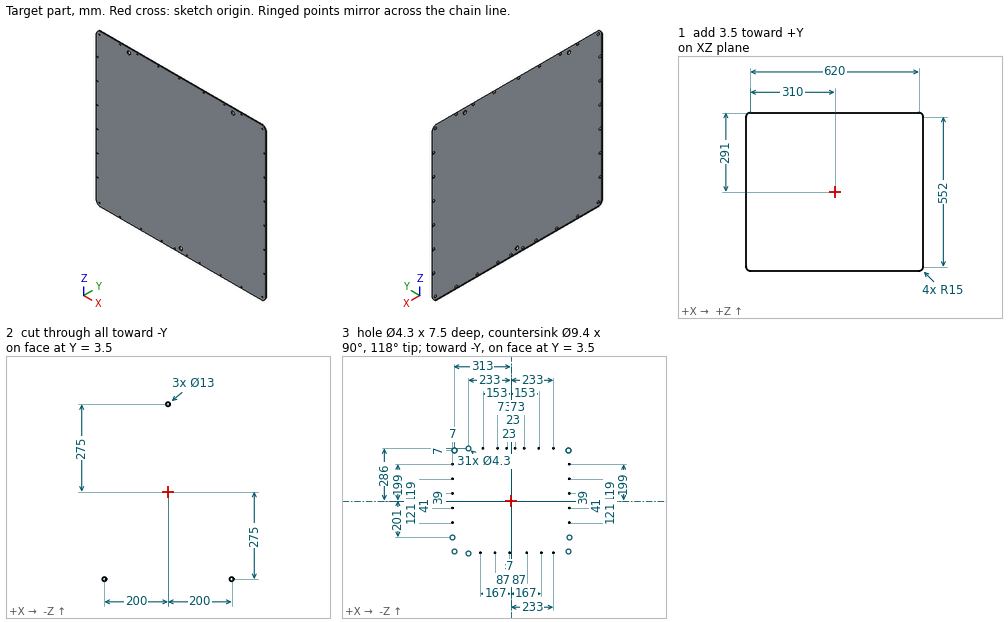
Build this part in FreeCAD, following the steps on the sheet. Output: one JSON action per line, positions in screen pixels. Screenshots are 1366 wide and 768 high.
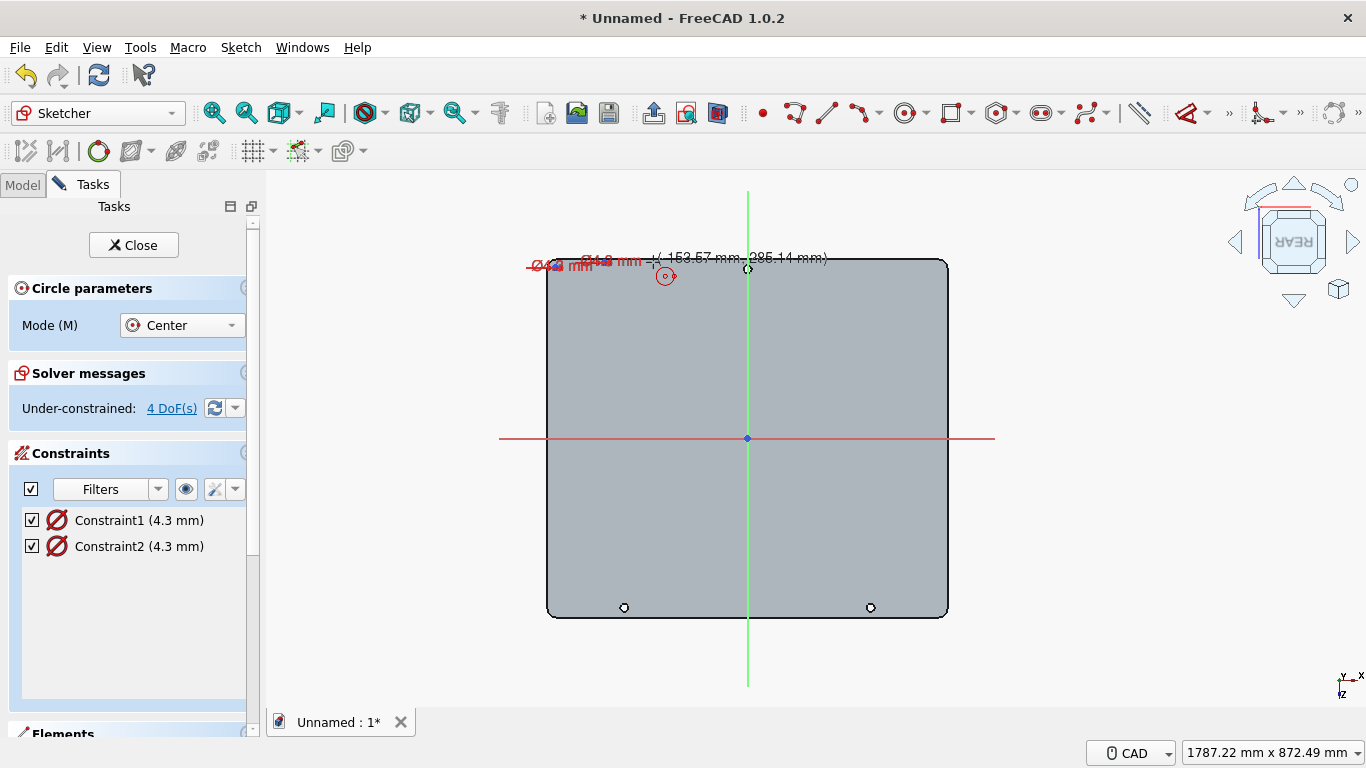
{"action": "left_click", "coordinate": [653, 262]}
{"action": "mouse_move", "coordinate": [654, 262]}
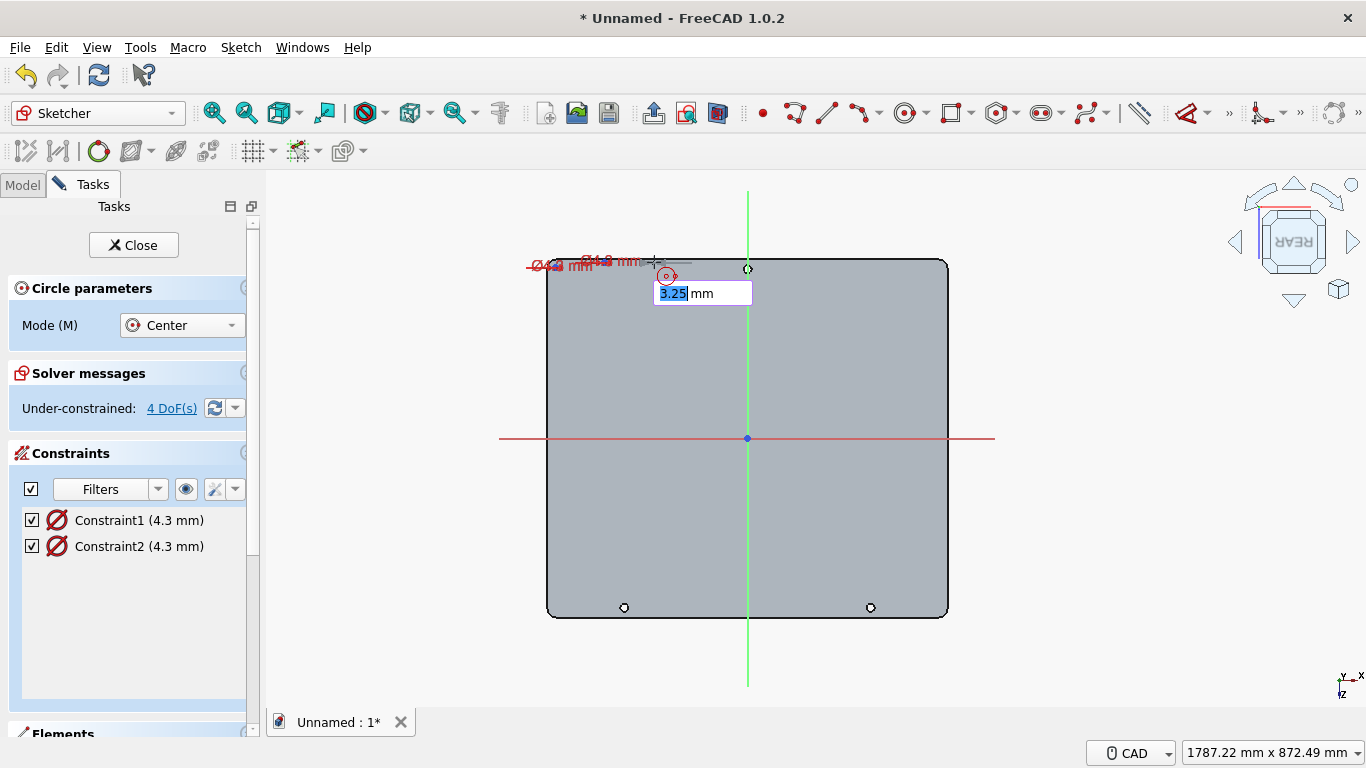
{"action": "type", "text": "4.3"}
{"action": "key", "text": "Return"}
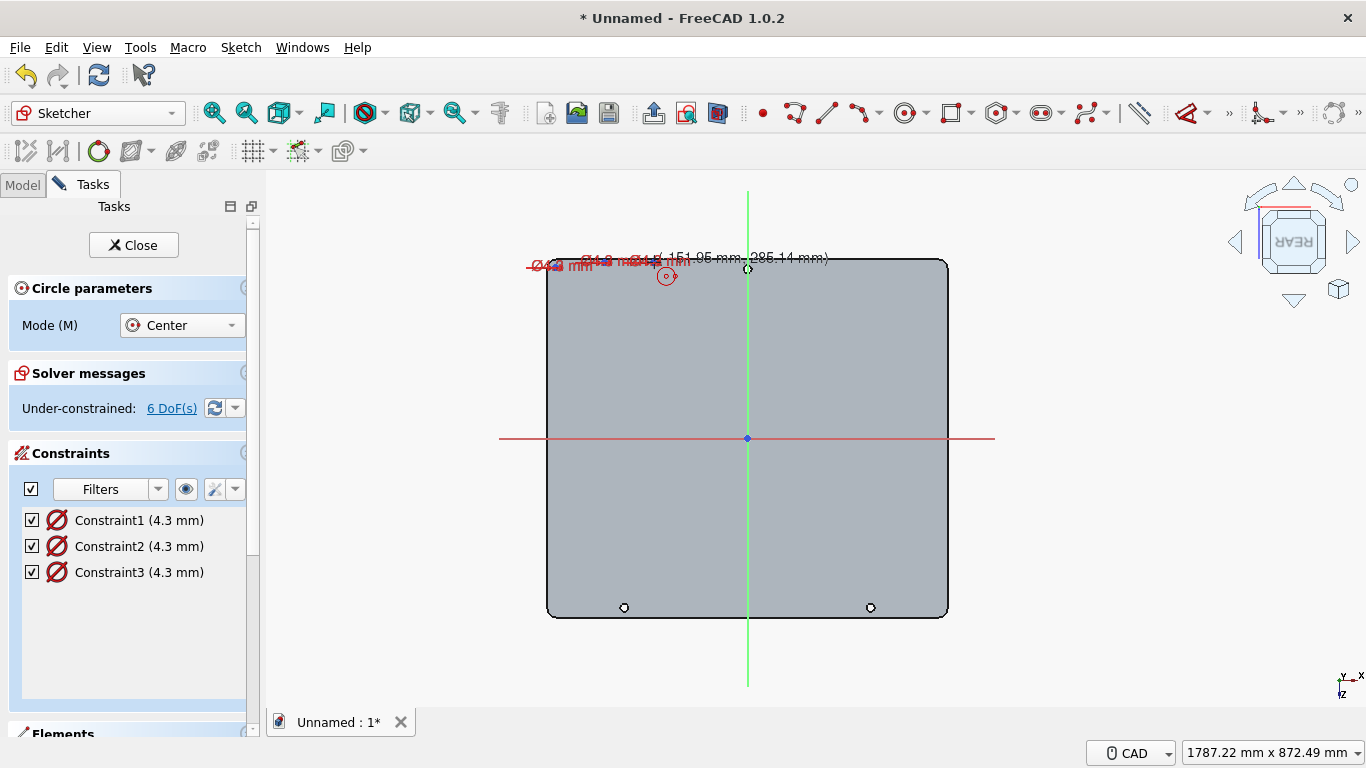
{"action": "scroll", "coordinate": [703, 262], "scroll_direction": "up", "scroll_amount": 15}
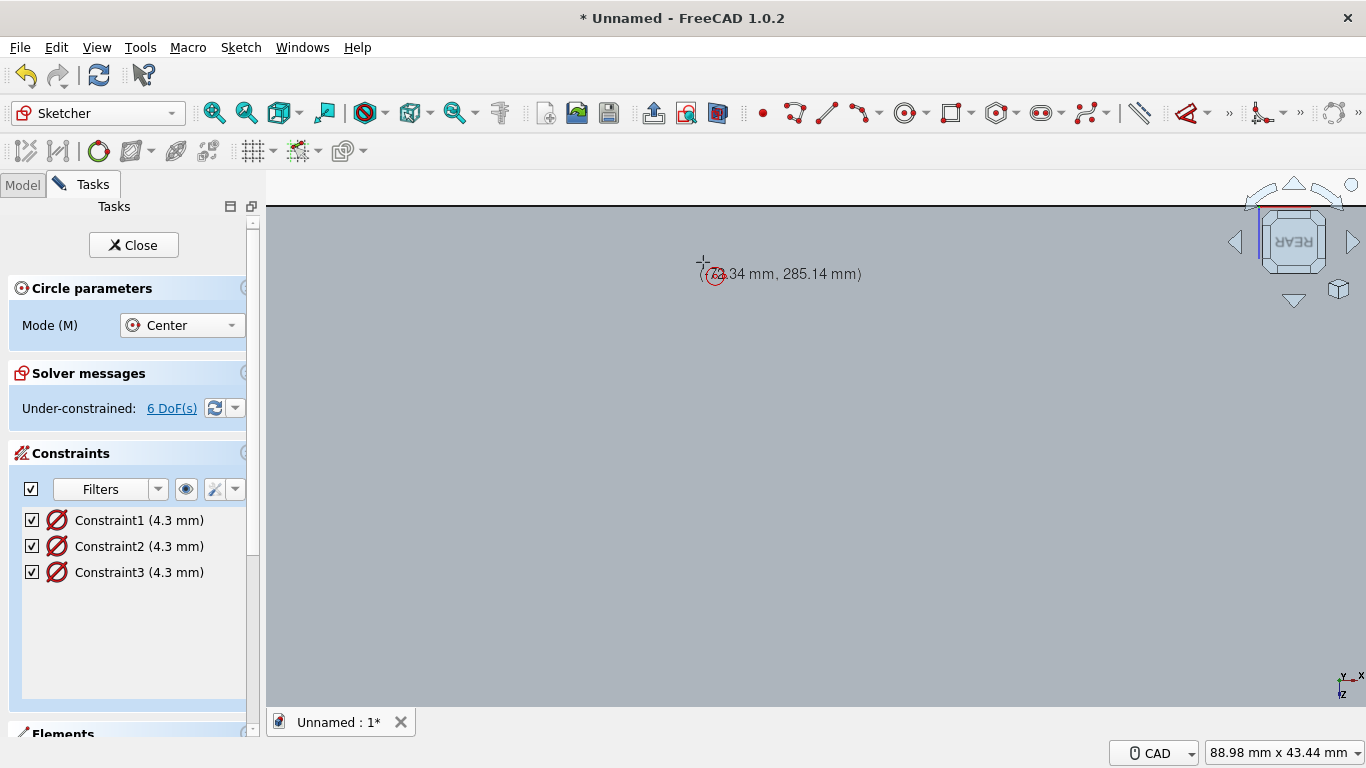
{"action": "scroll", "coordinate": [703, 262], "scroll_direction": "down", "scroll_amount": 15}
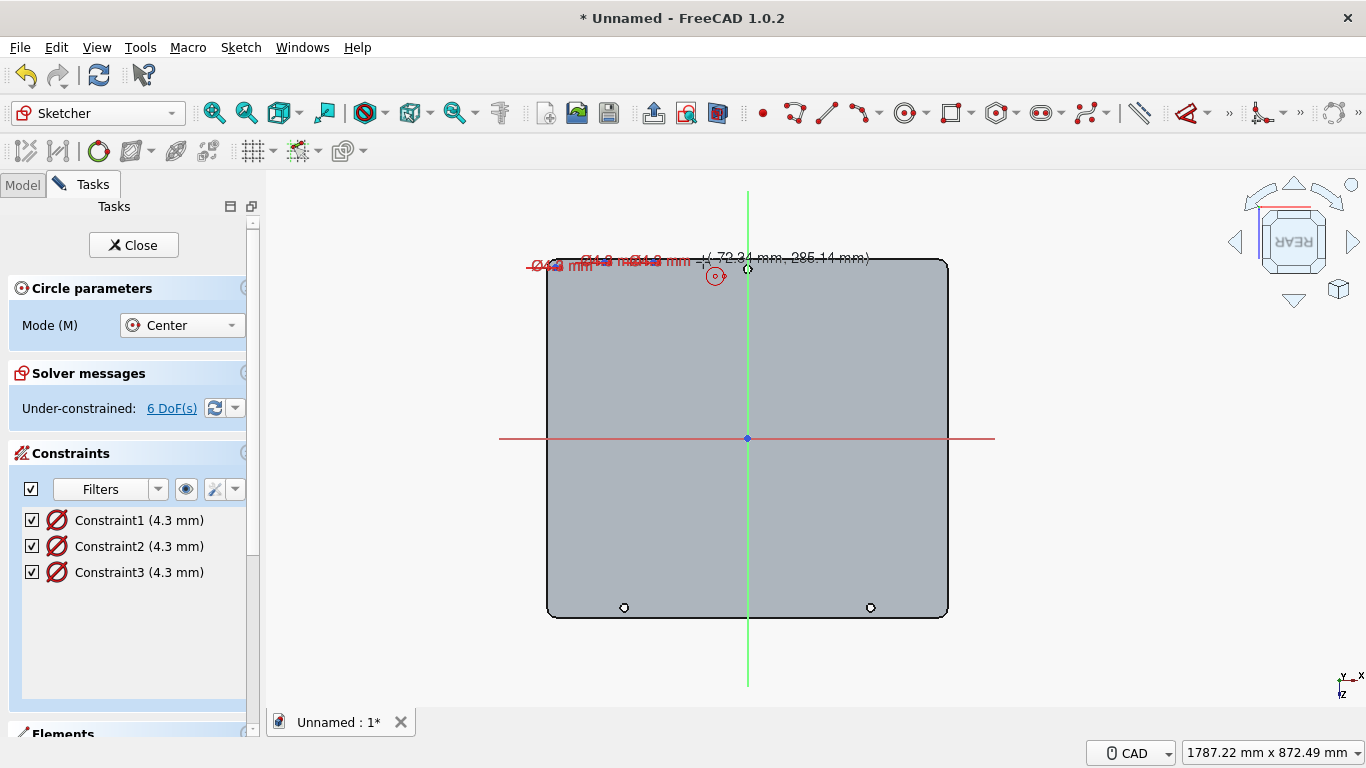
{"action": "left_click", "coordinate": [703, 262]}
{"action": "mouse_move", "coordinate": [704, 262]}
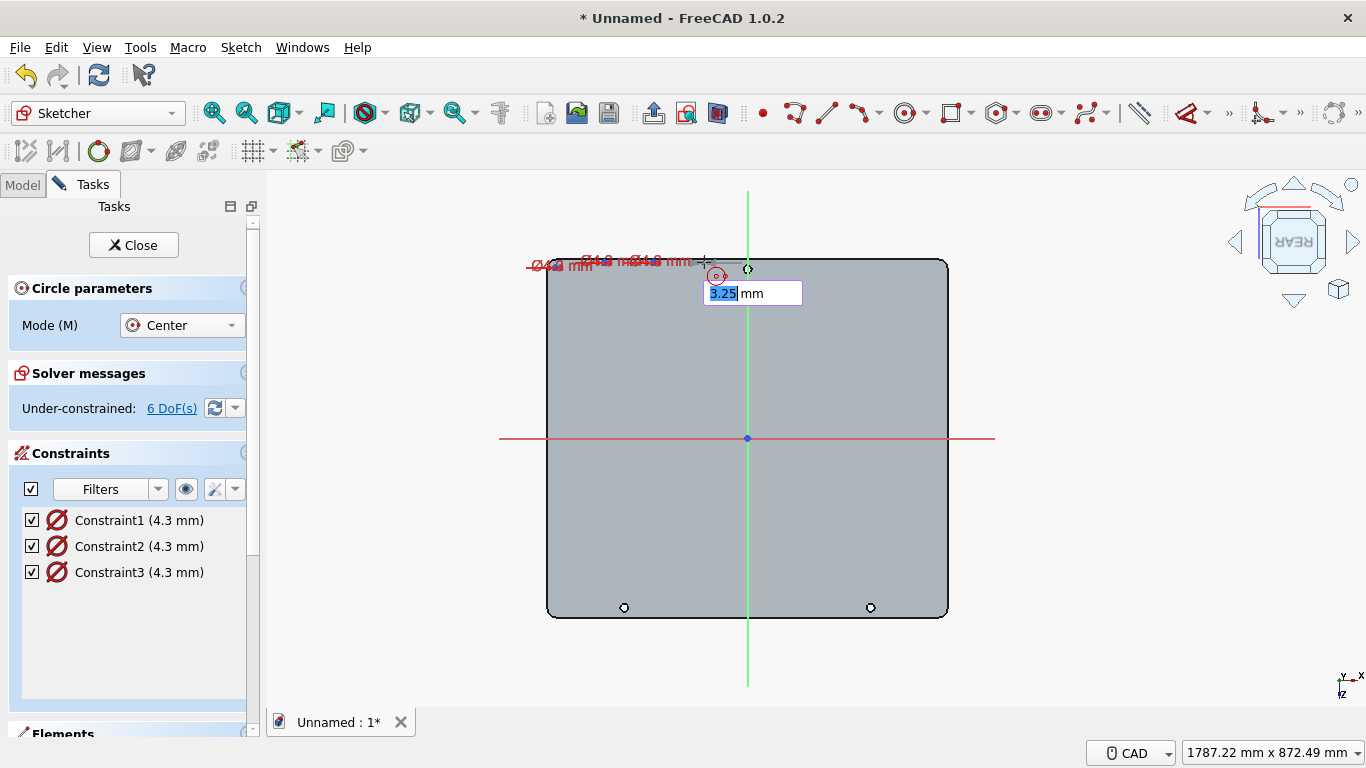
{"action": "type", "text": "4.3"}
{"action": "key", "text": "Return"}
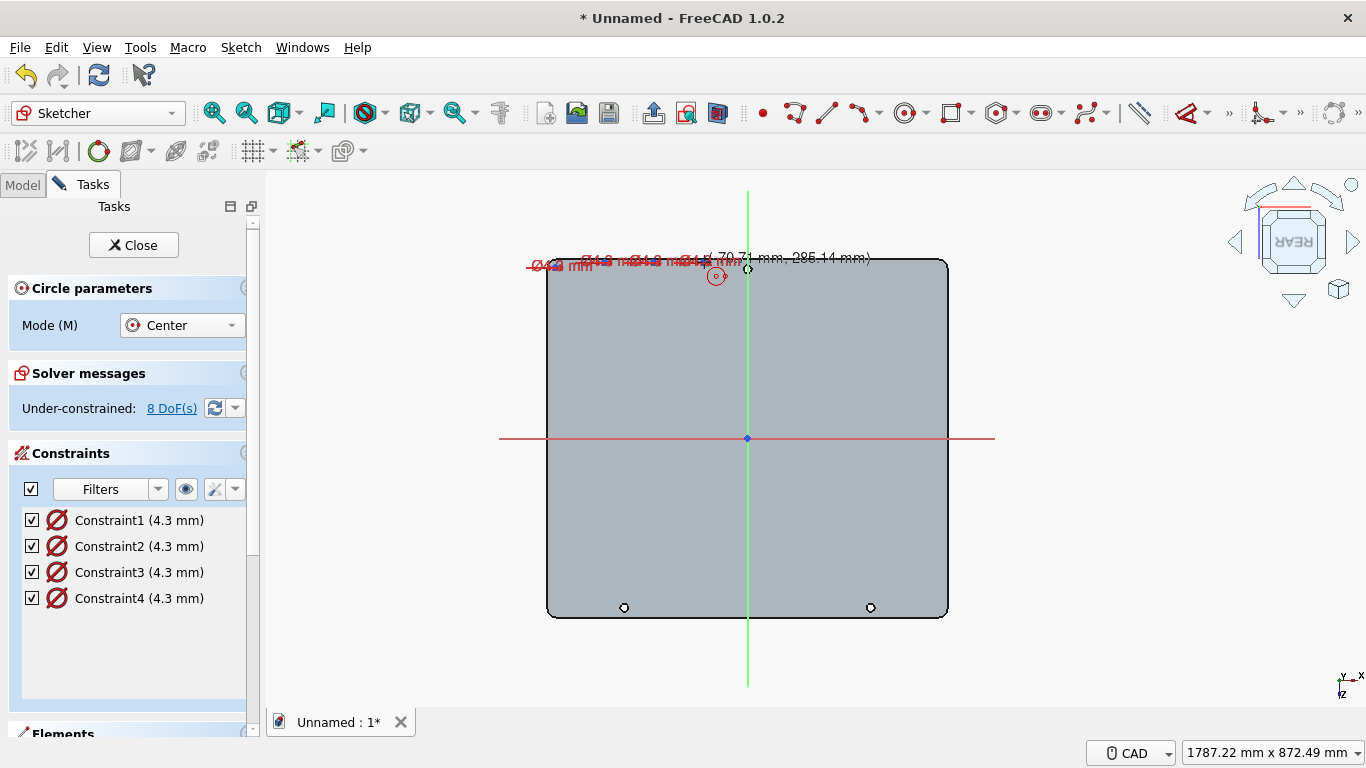
{"action": "scroll", "coordinate": [733, 262], "scroll_direction": "up", "scroll_amount": 15}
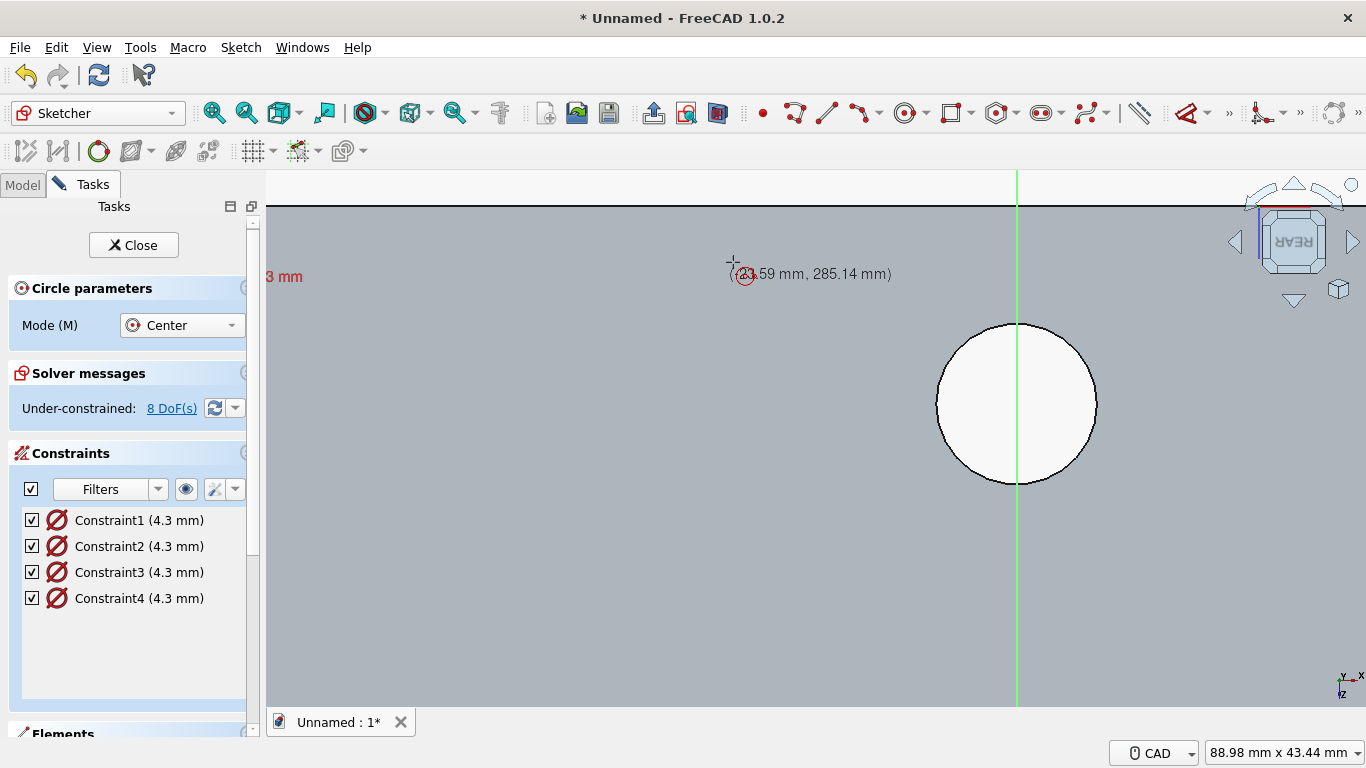
{"action": "scroll", "coordinate": [733, 262], "scroll_direction": "down", "scroll_amount": 15}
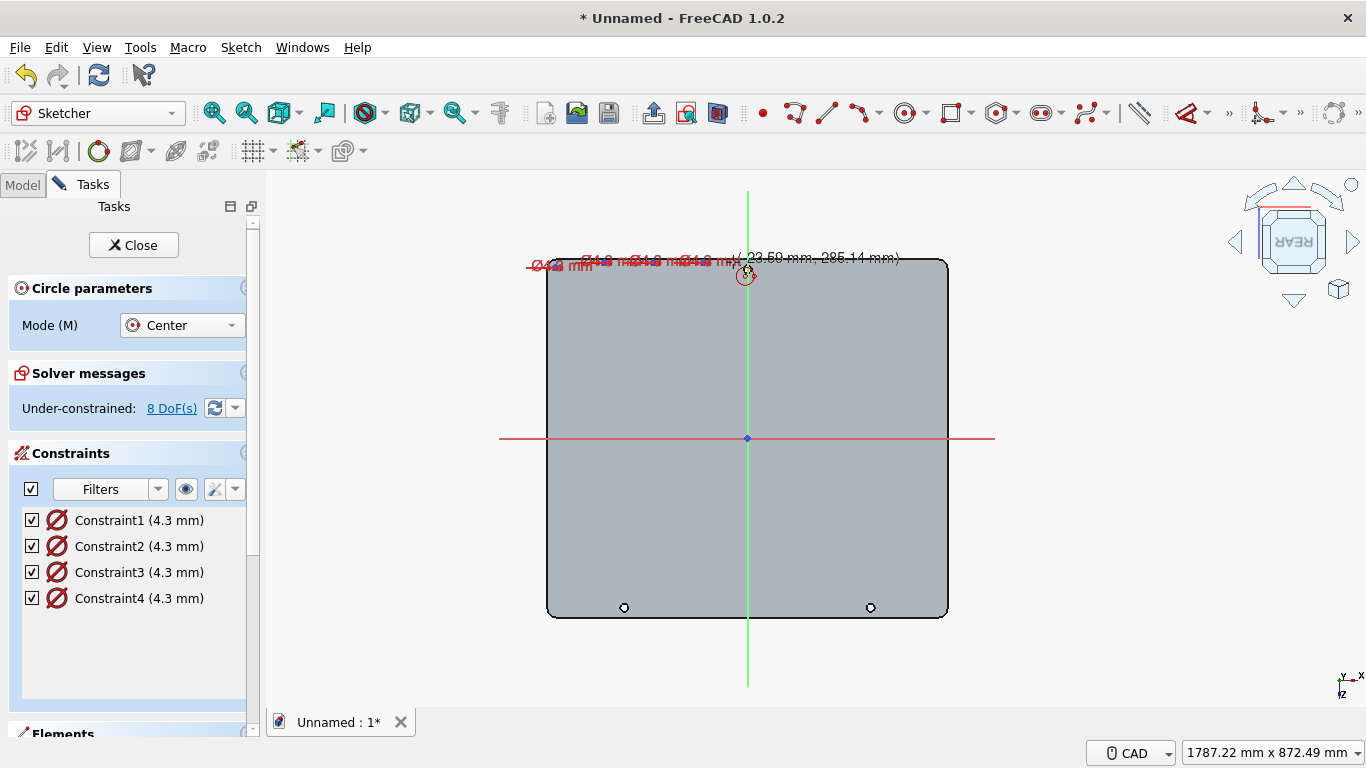
{"action": "left_click", "coordinate": [733, 262]}
{"action": "mouse_move", "coordinate": [732, 262]}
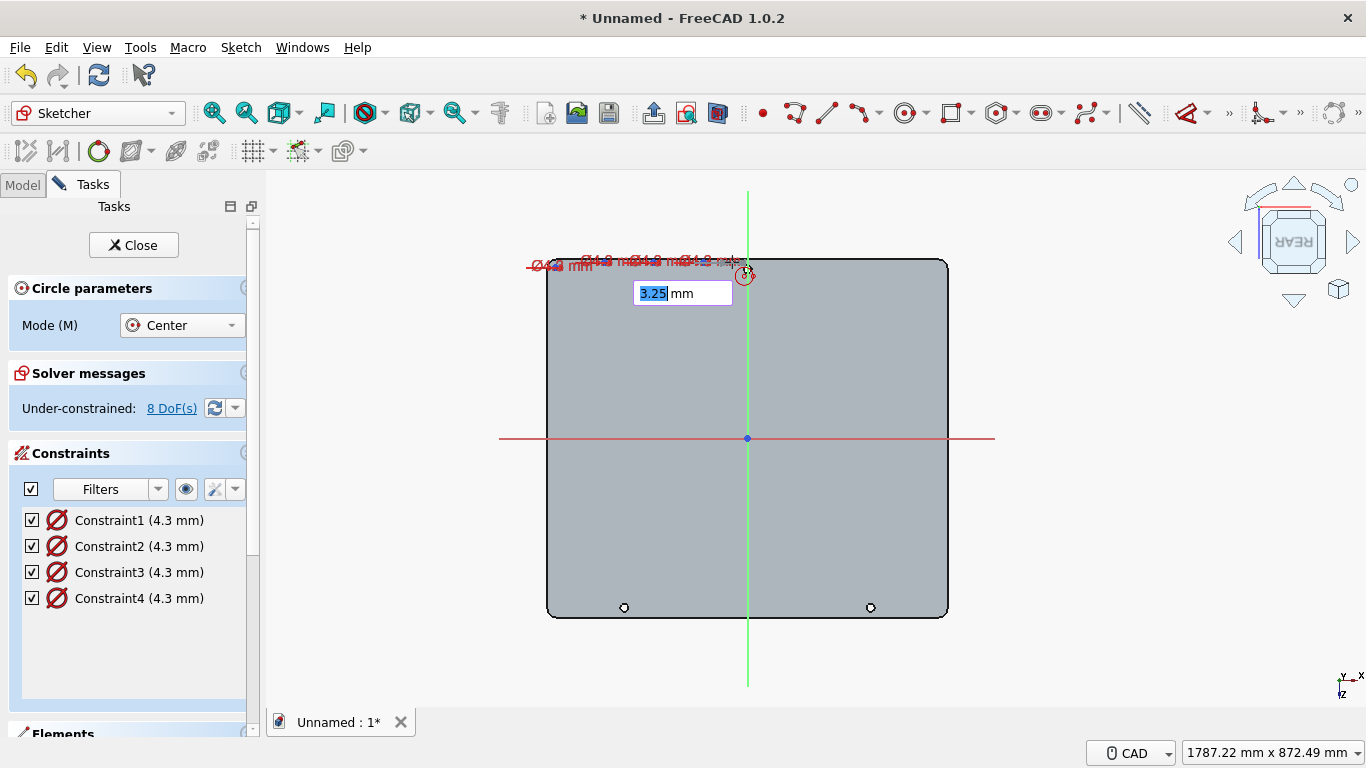
{"action": "type", "text": "4.3"}
{"action": "key", "text": "Return"}